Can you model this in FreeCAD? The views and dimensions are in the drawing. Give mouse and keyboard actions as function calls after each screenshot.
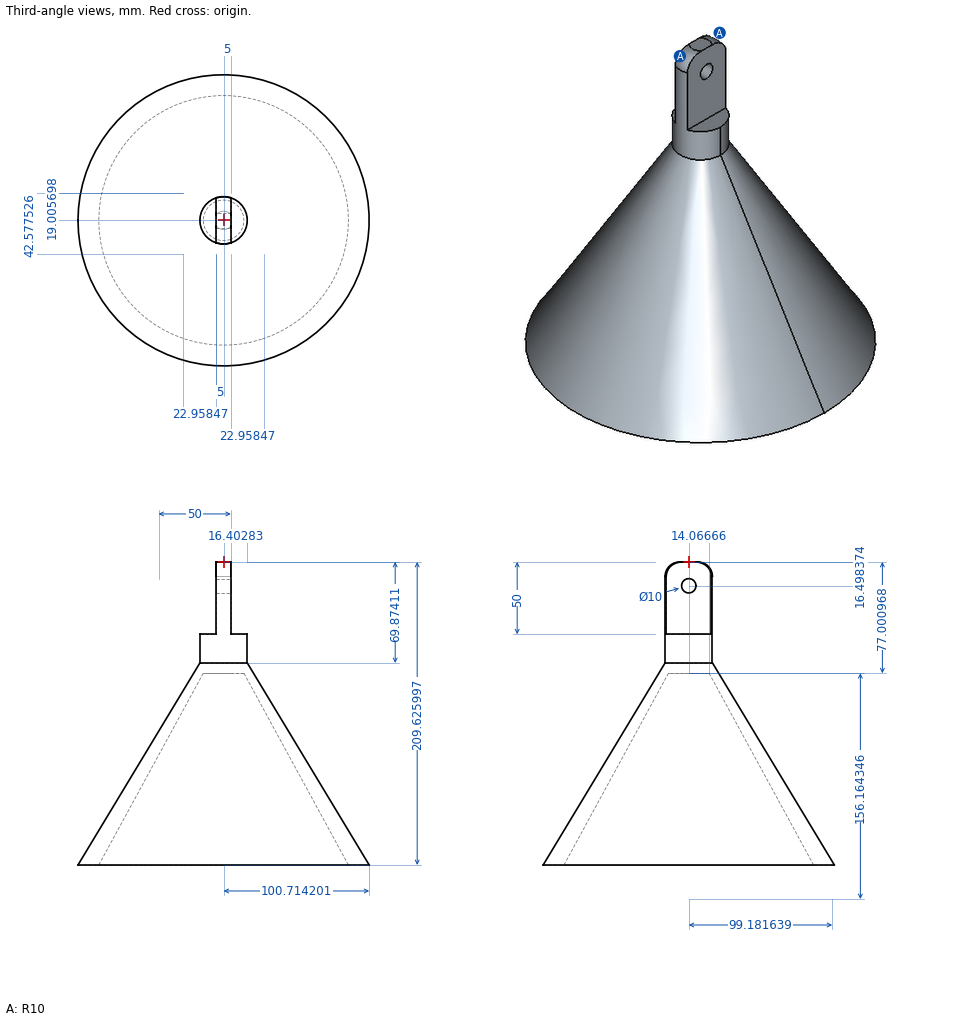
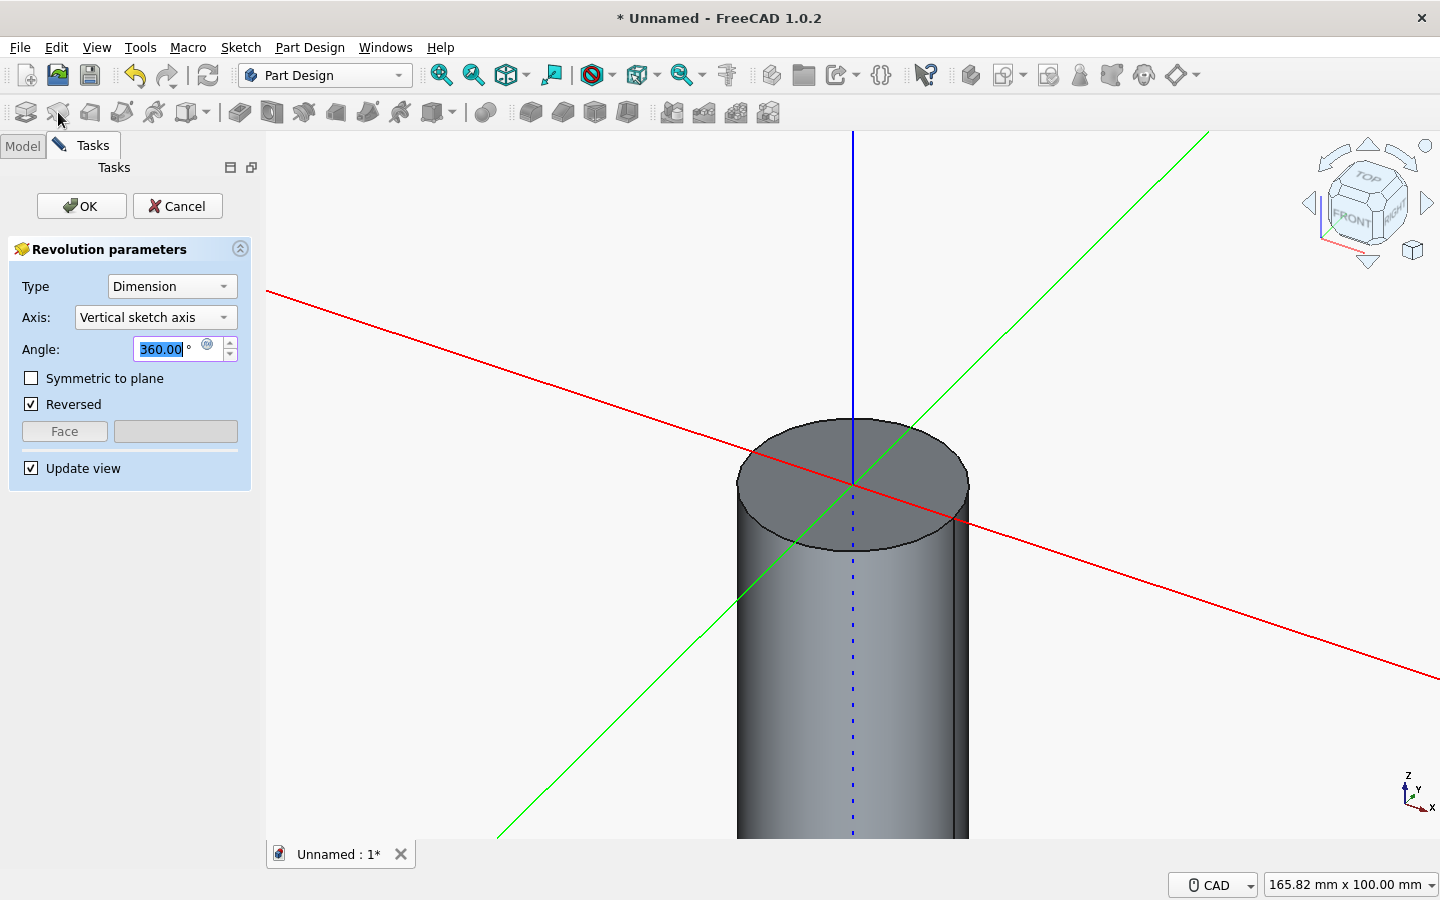
click(82, 206)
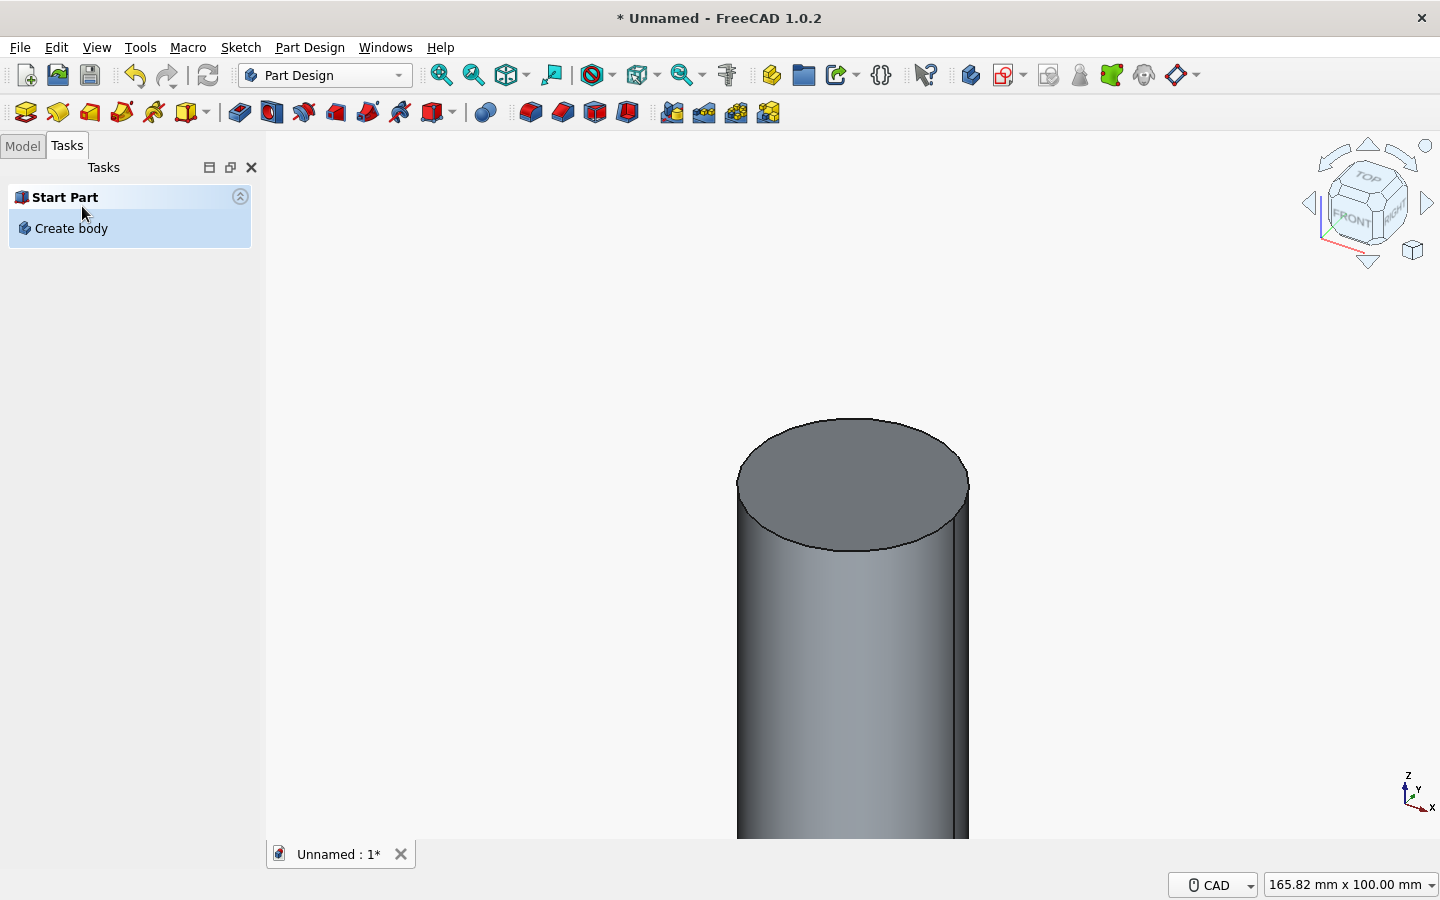
click(442, 76)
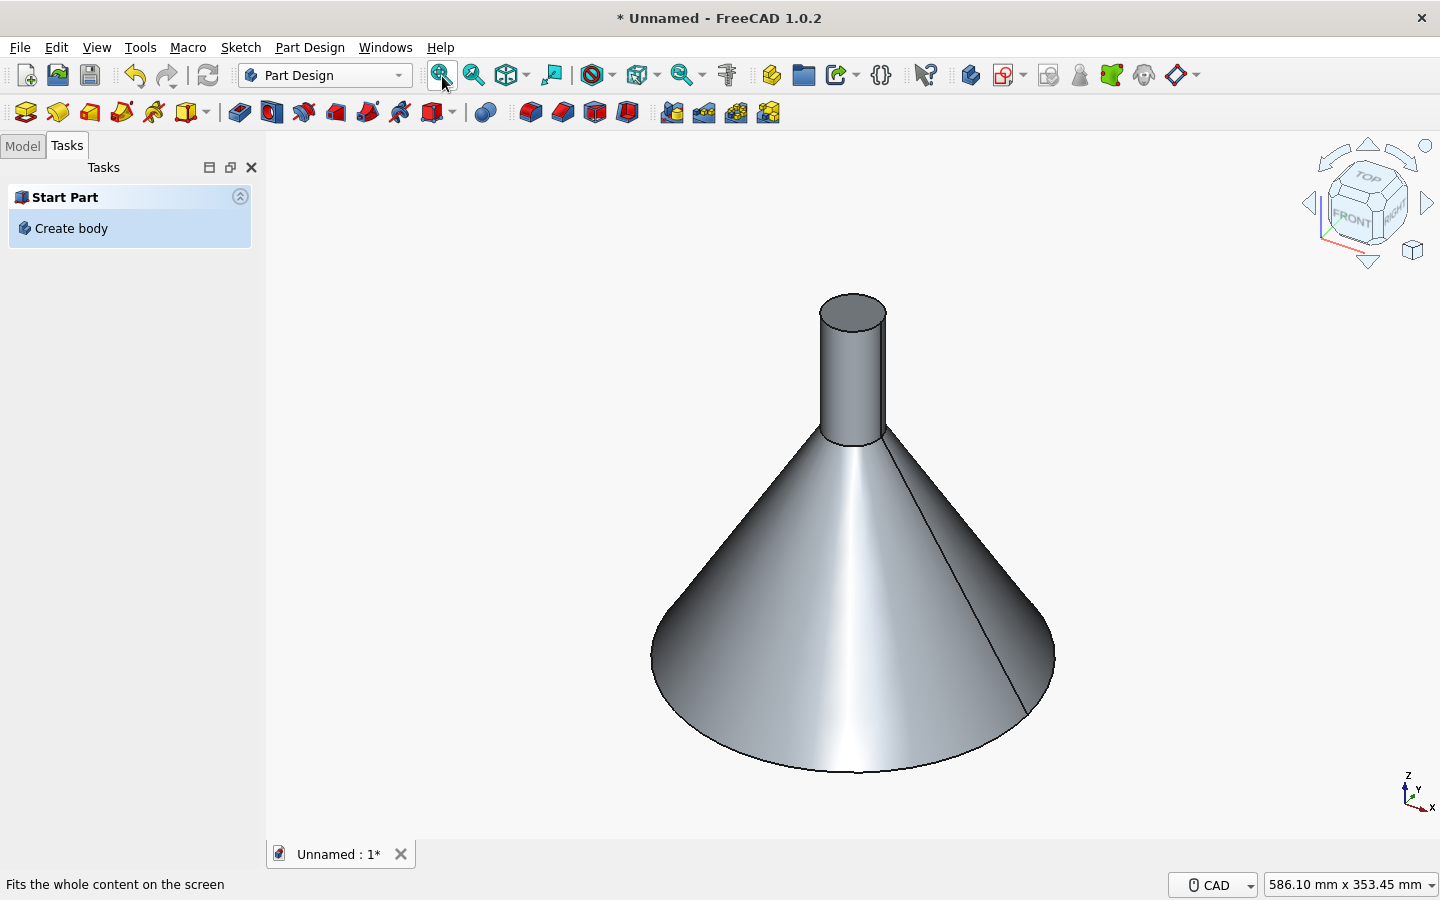
click(1004, 76)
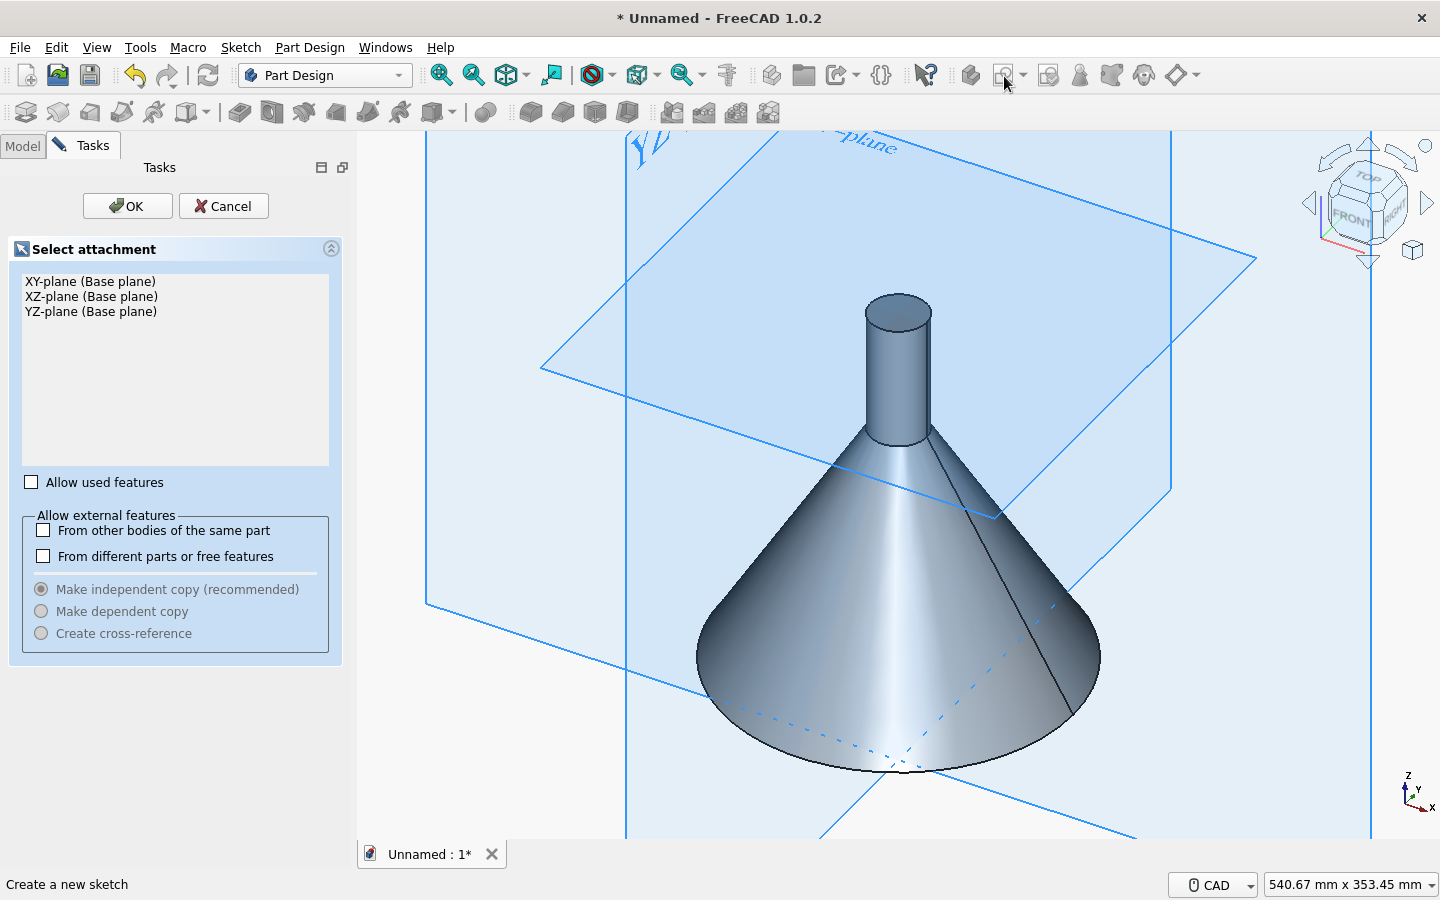
click(82, 282)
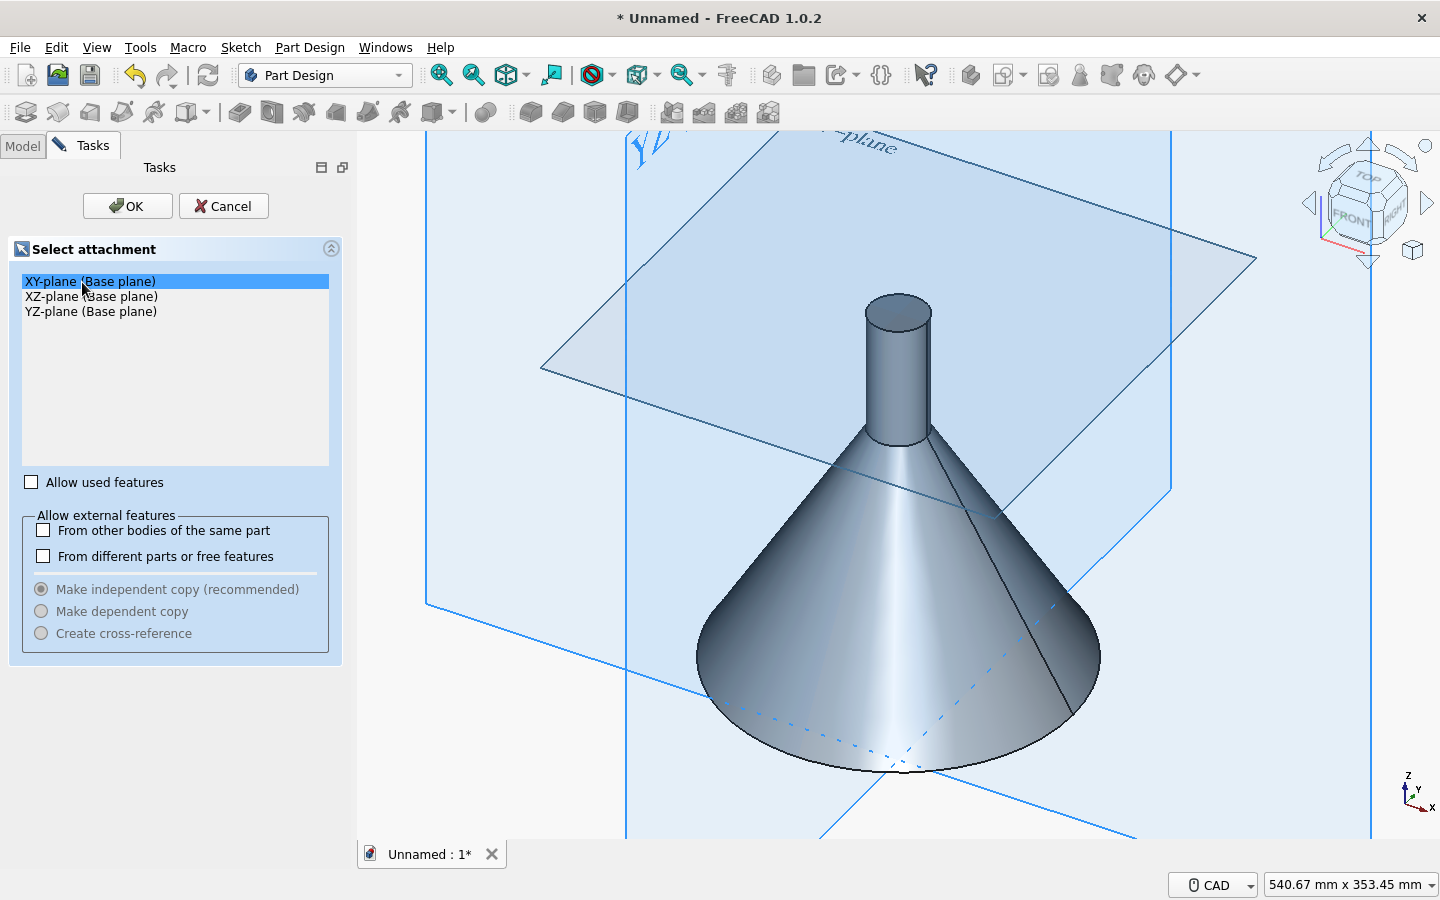
click(128, 206)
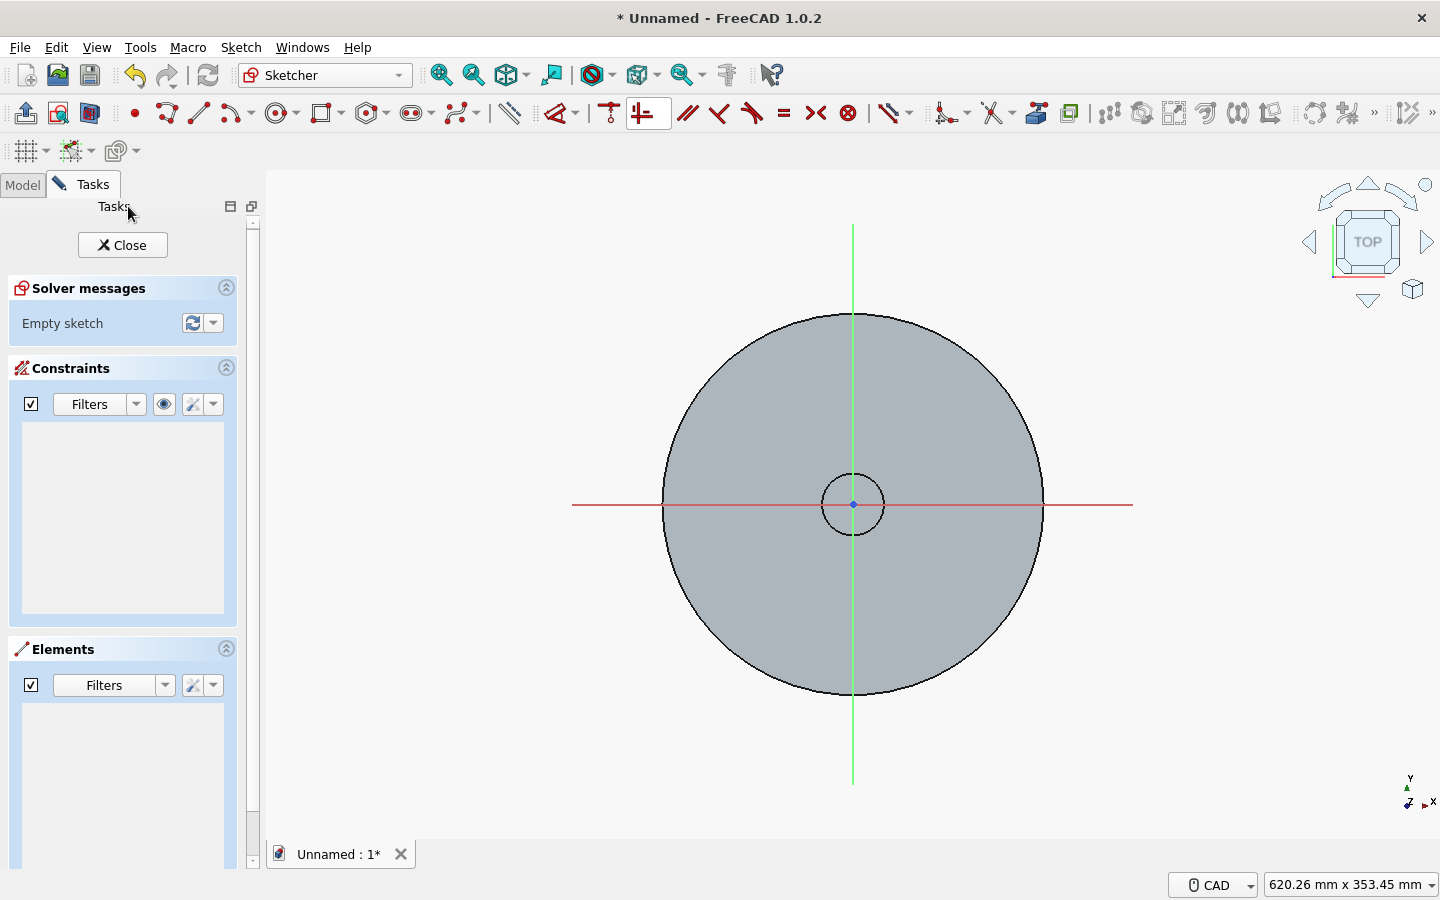
scroll(870, 510, up, 8)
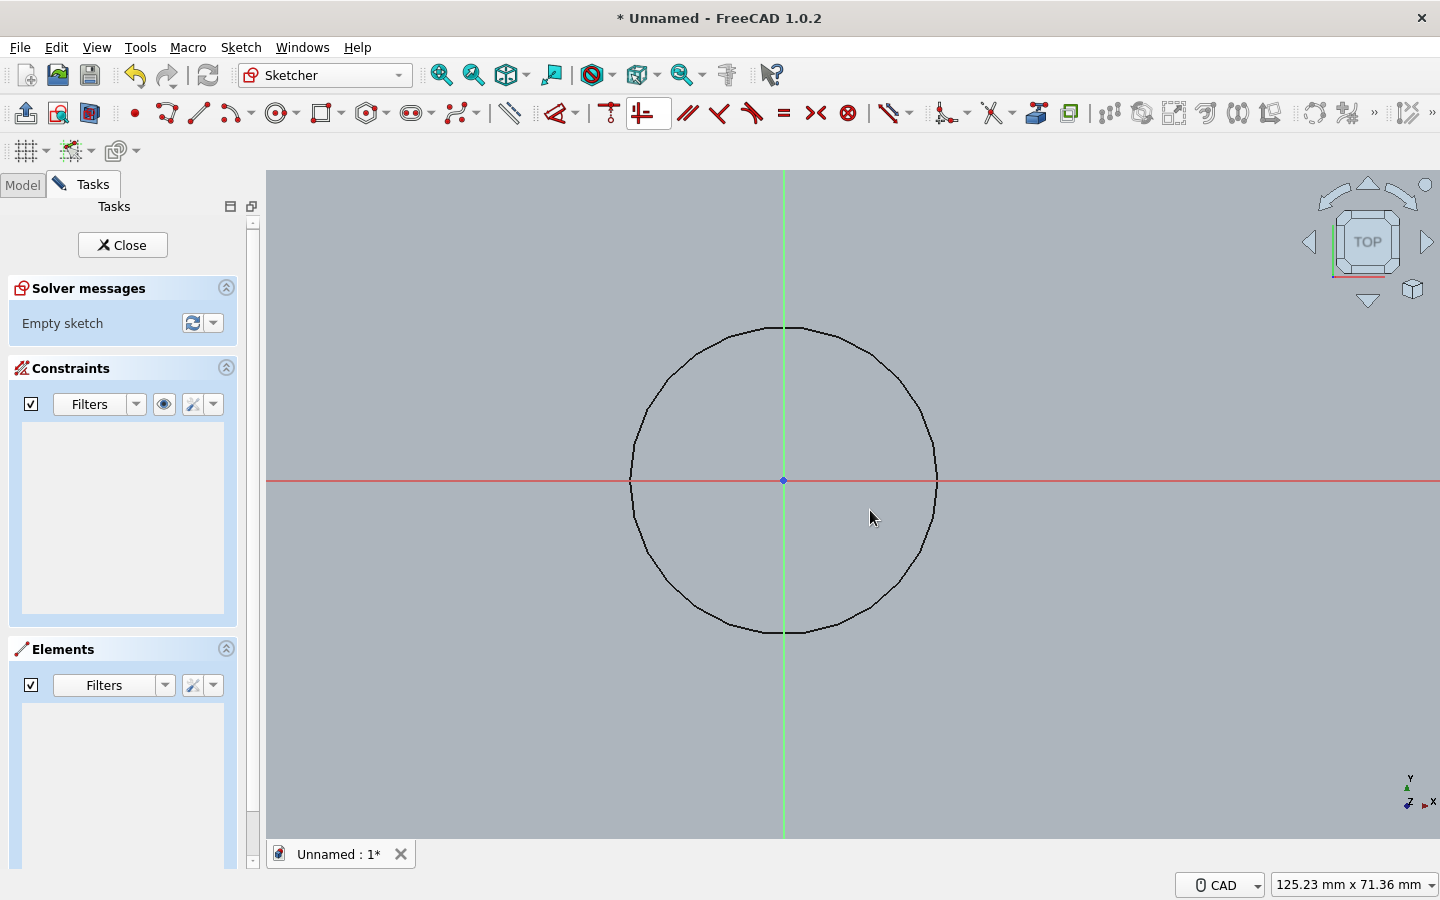
click(322, 114)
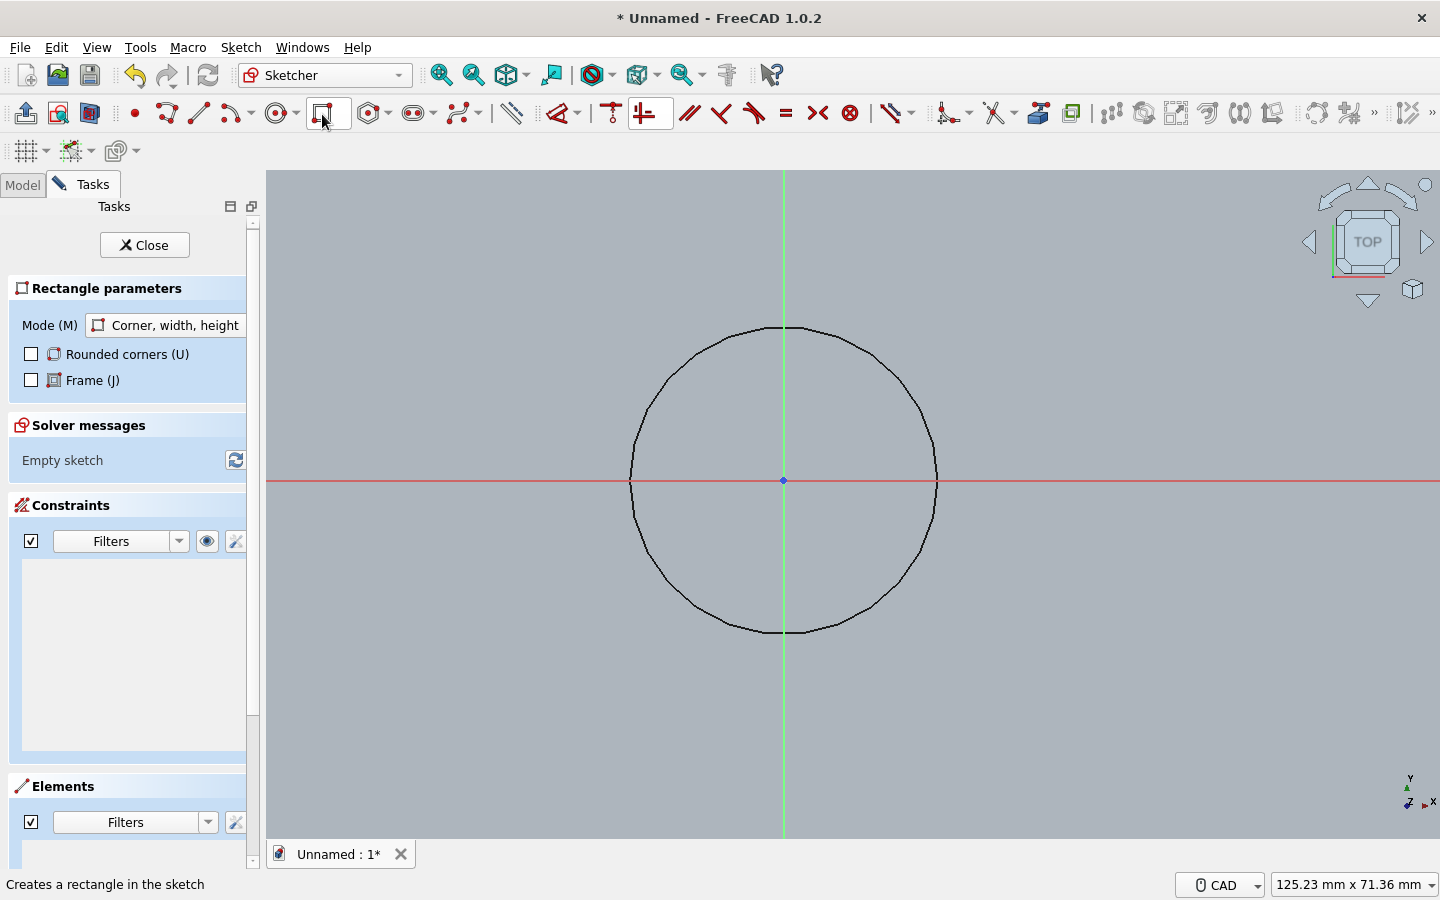
click(522, 303)
click(737, 702)